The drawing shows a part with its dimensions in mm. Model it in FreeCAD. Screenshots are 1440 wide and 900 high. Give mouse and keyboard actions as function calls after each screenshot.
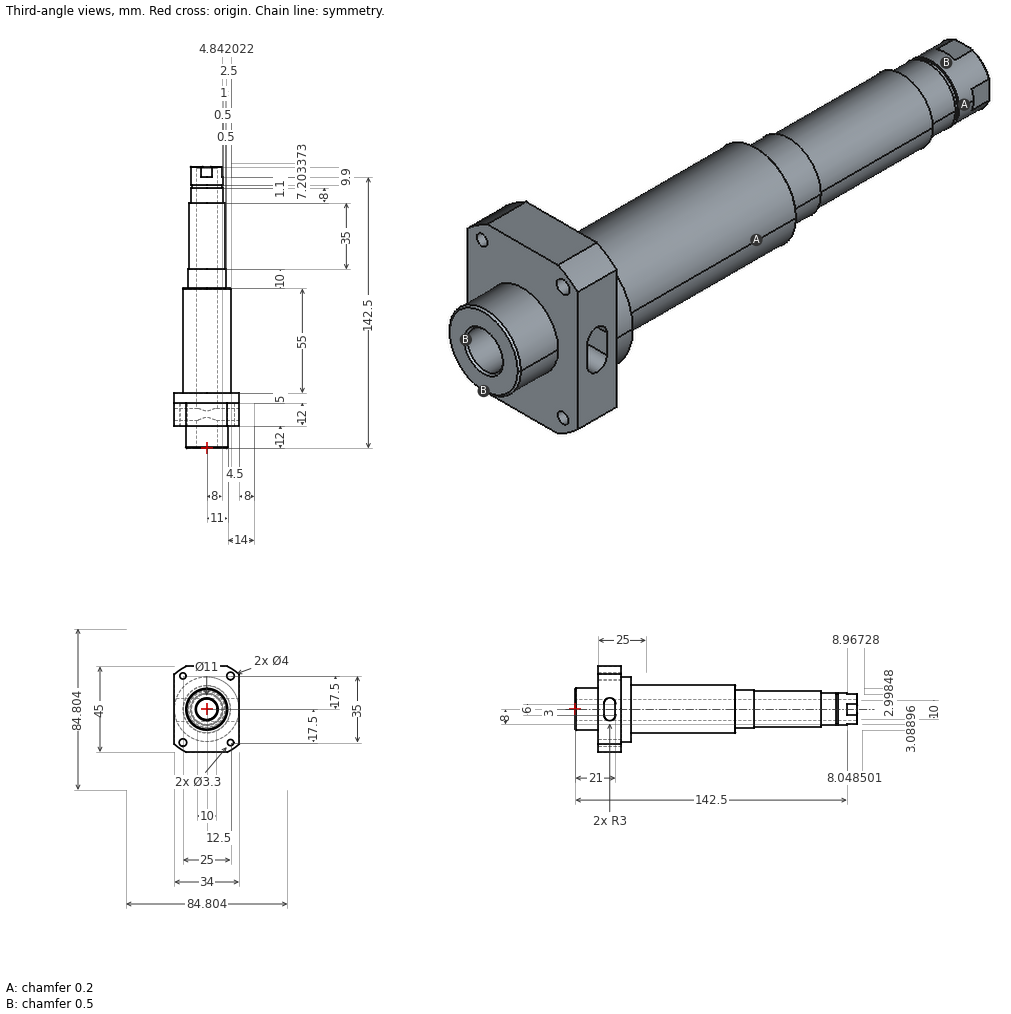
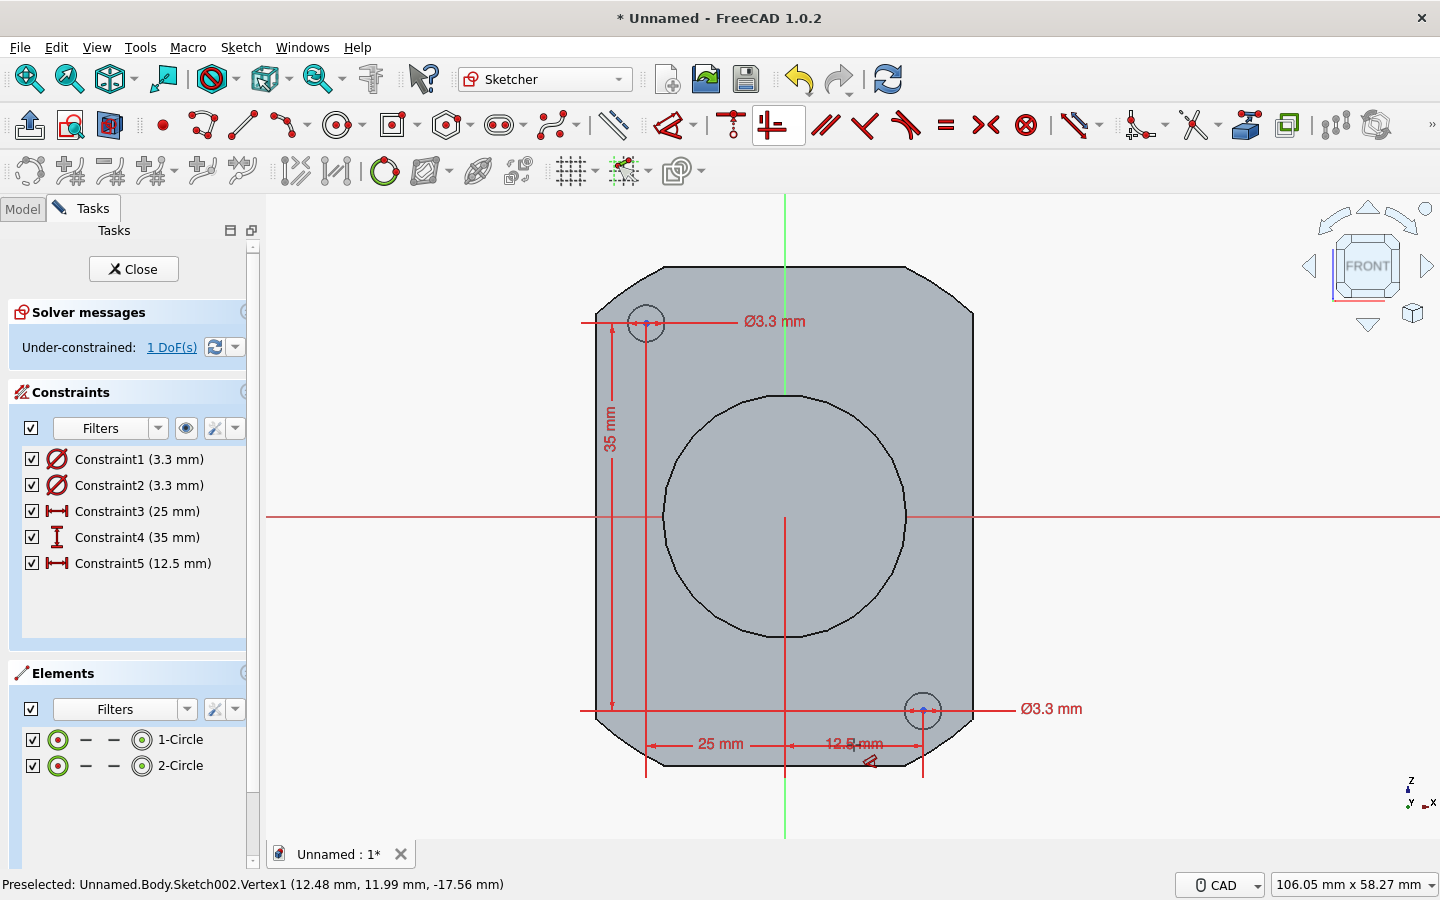
click(923, 711)
click(957, 614)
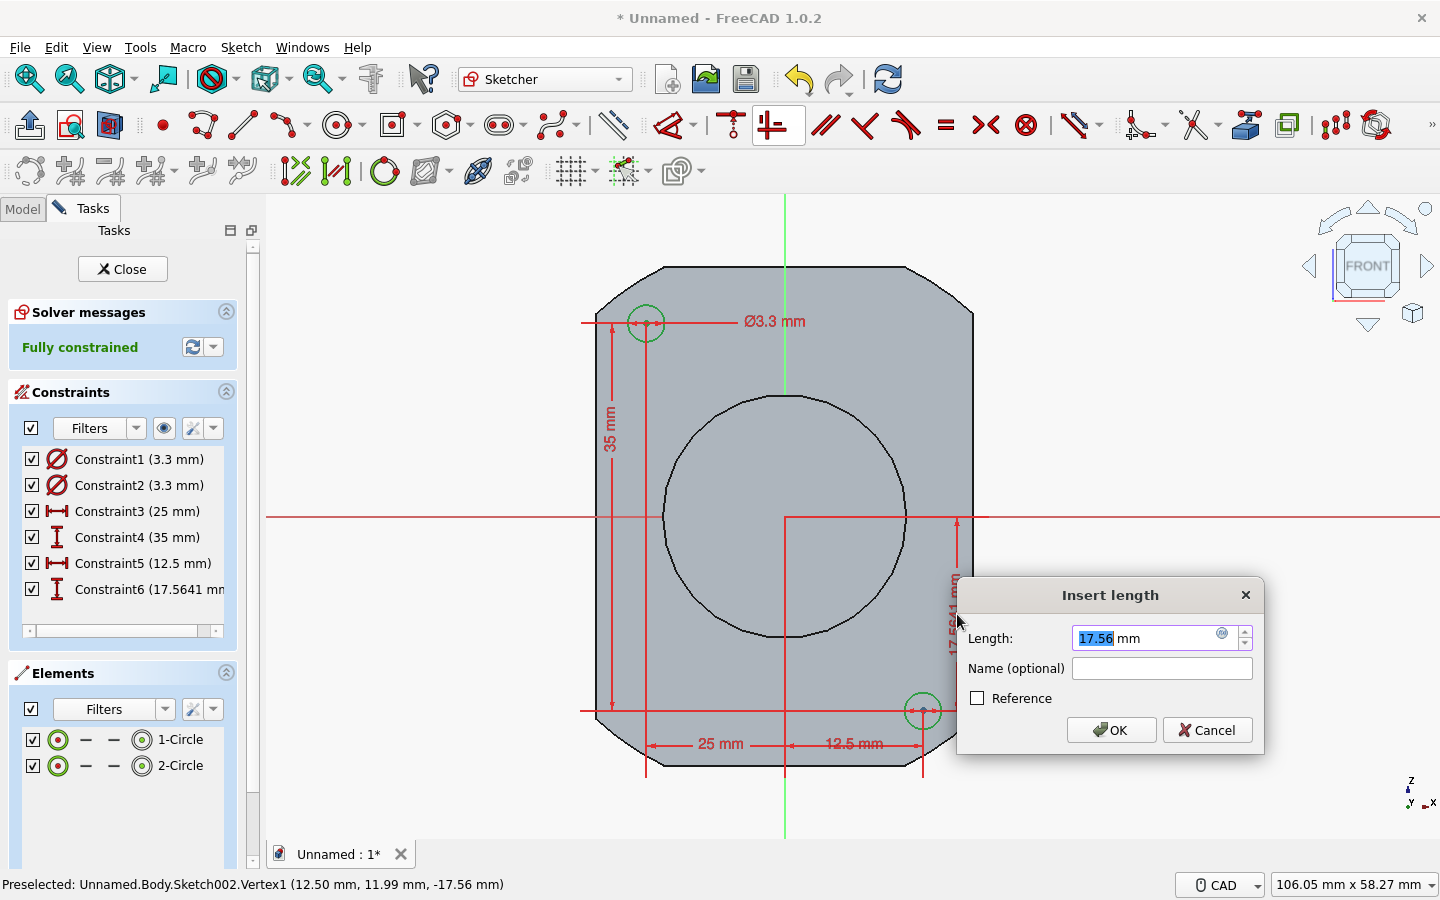
text(17.5)
key(Return)
key(Escape)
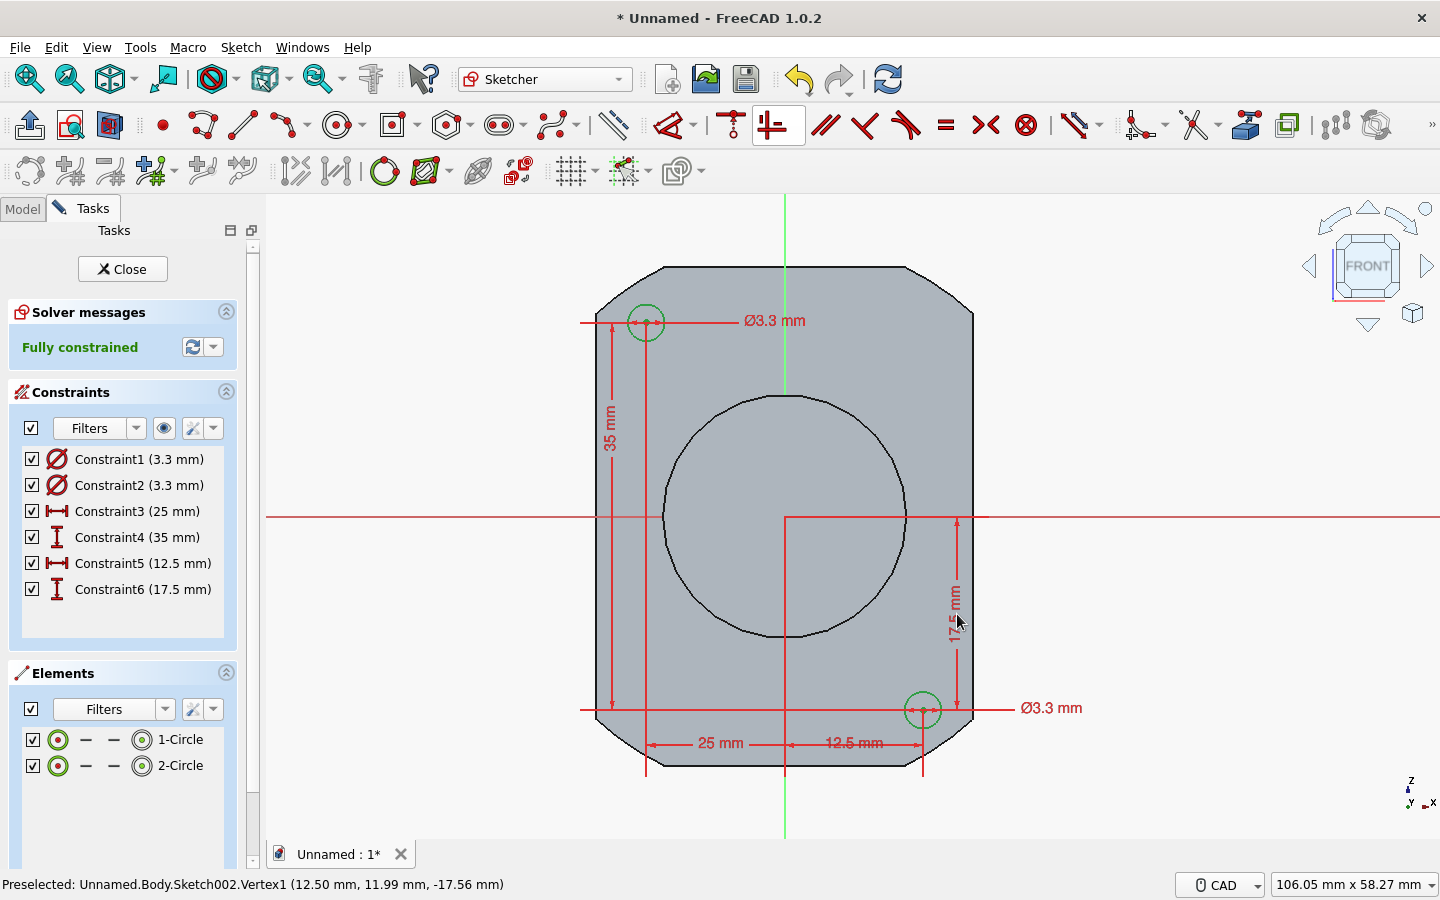
click(123, 269)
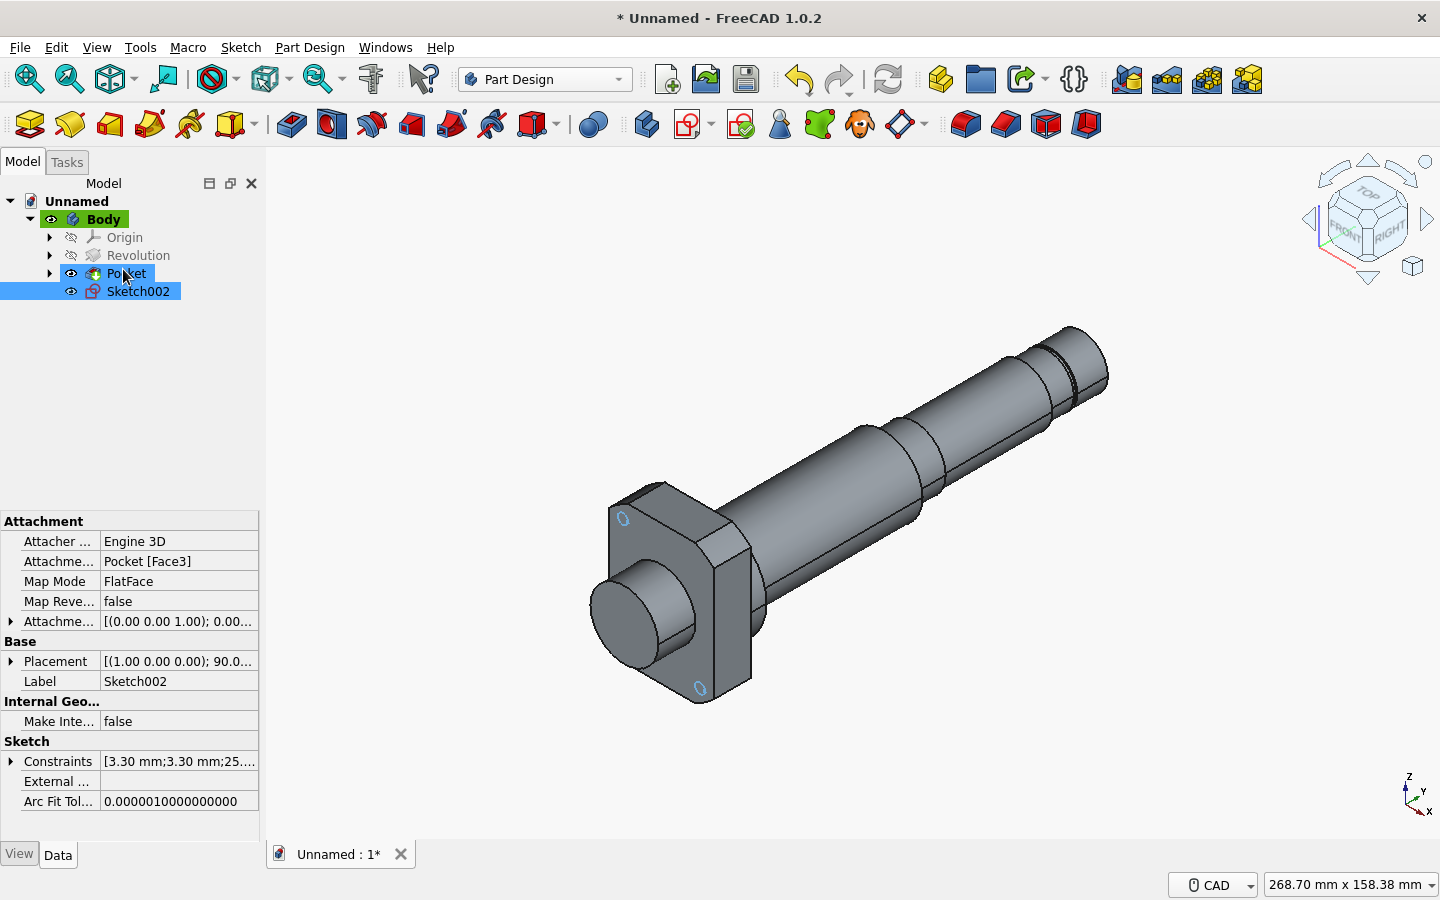
click(292, 124)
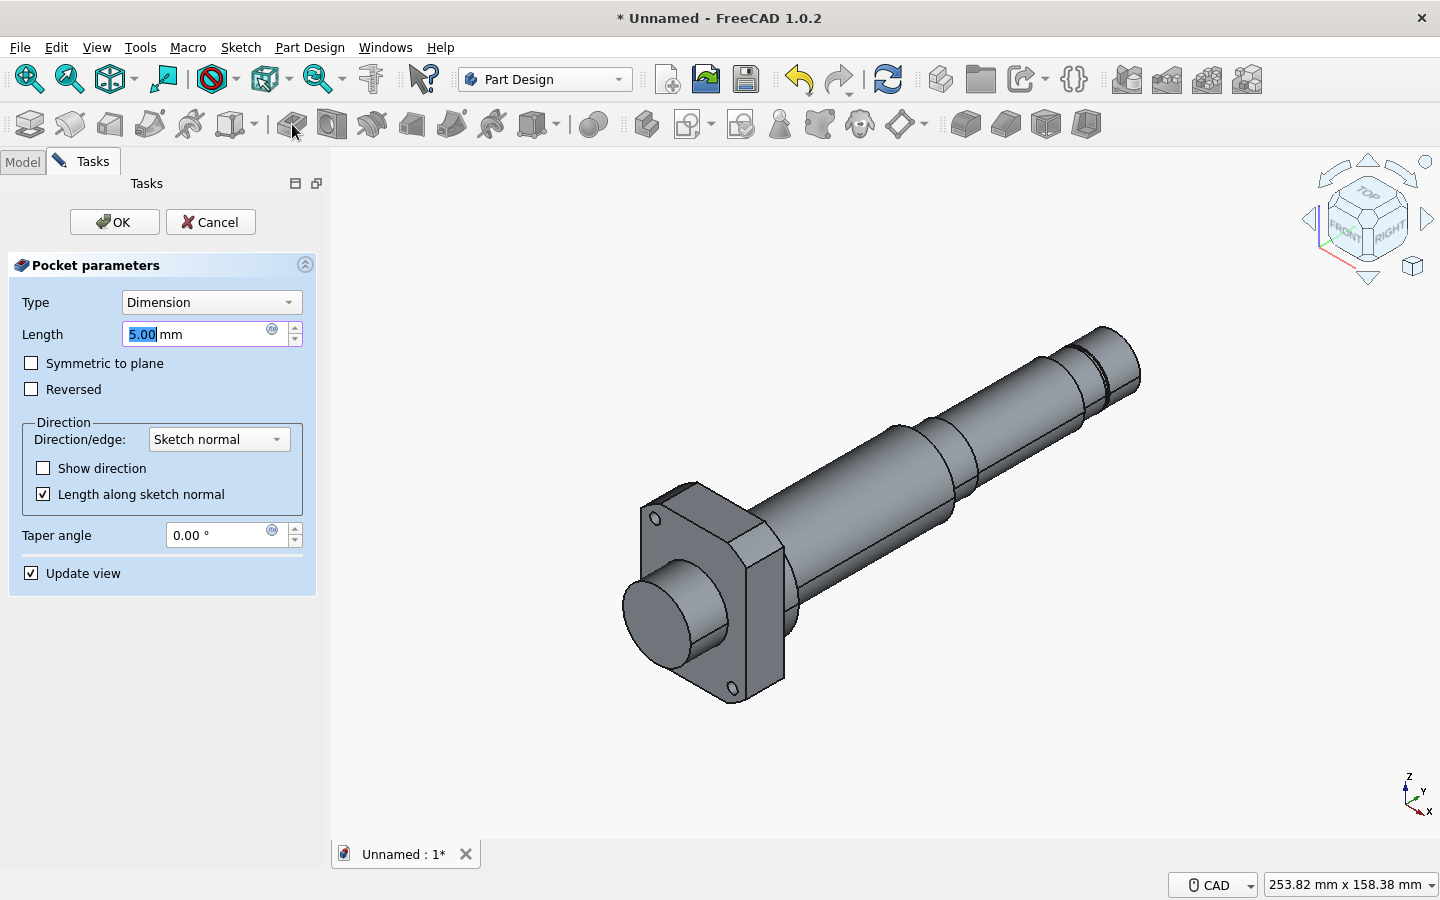
click(212, 302)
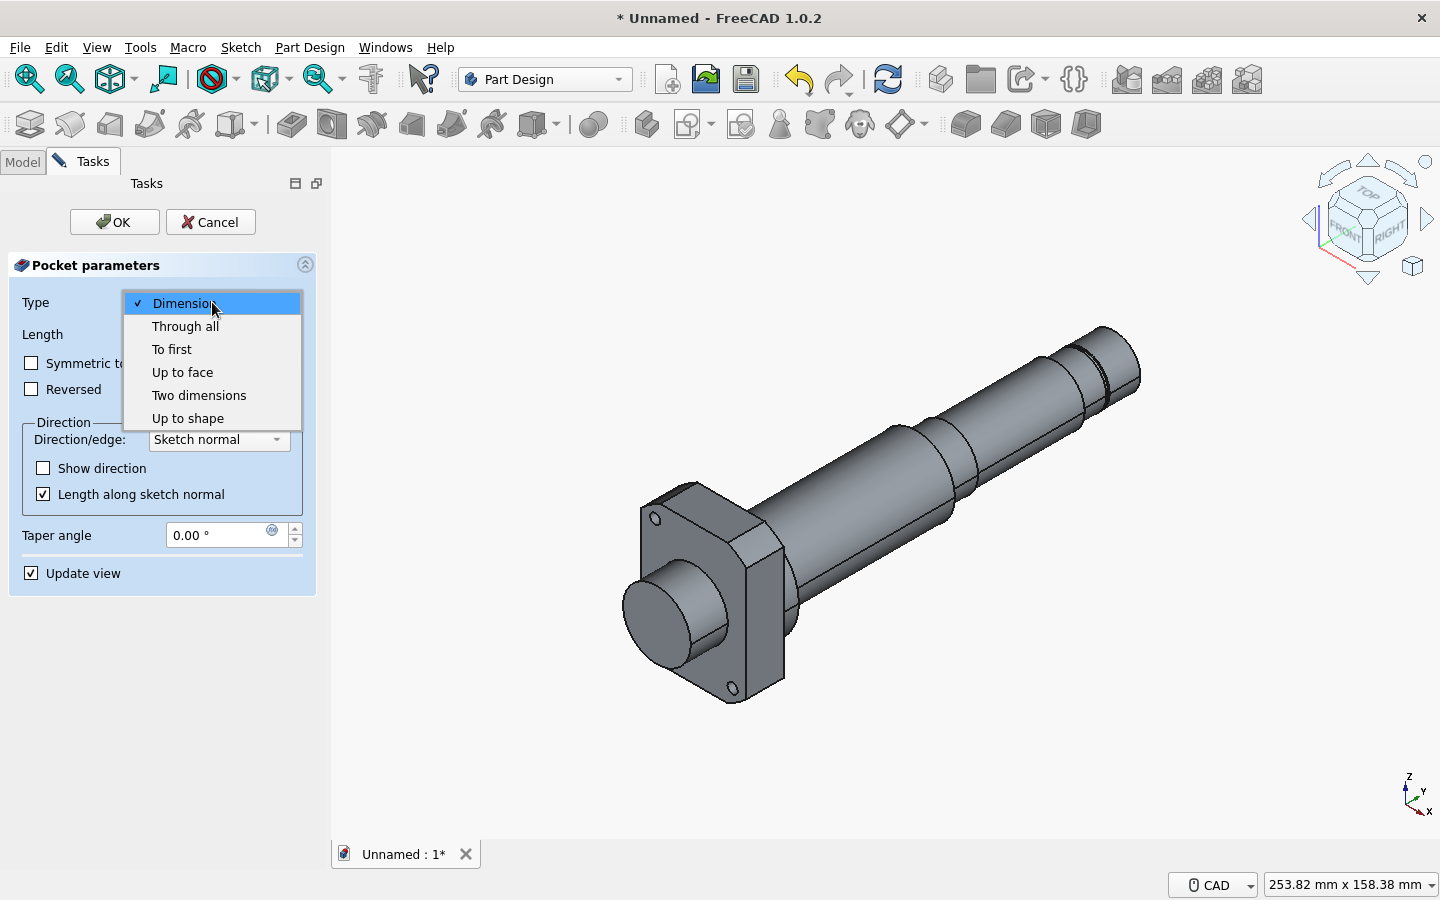
click(212, 326)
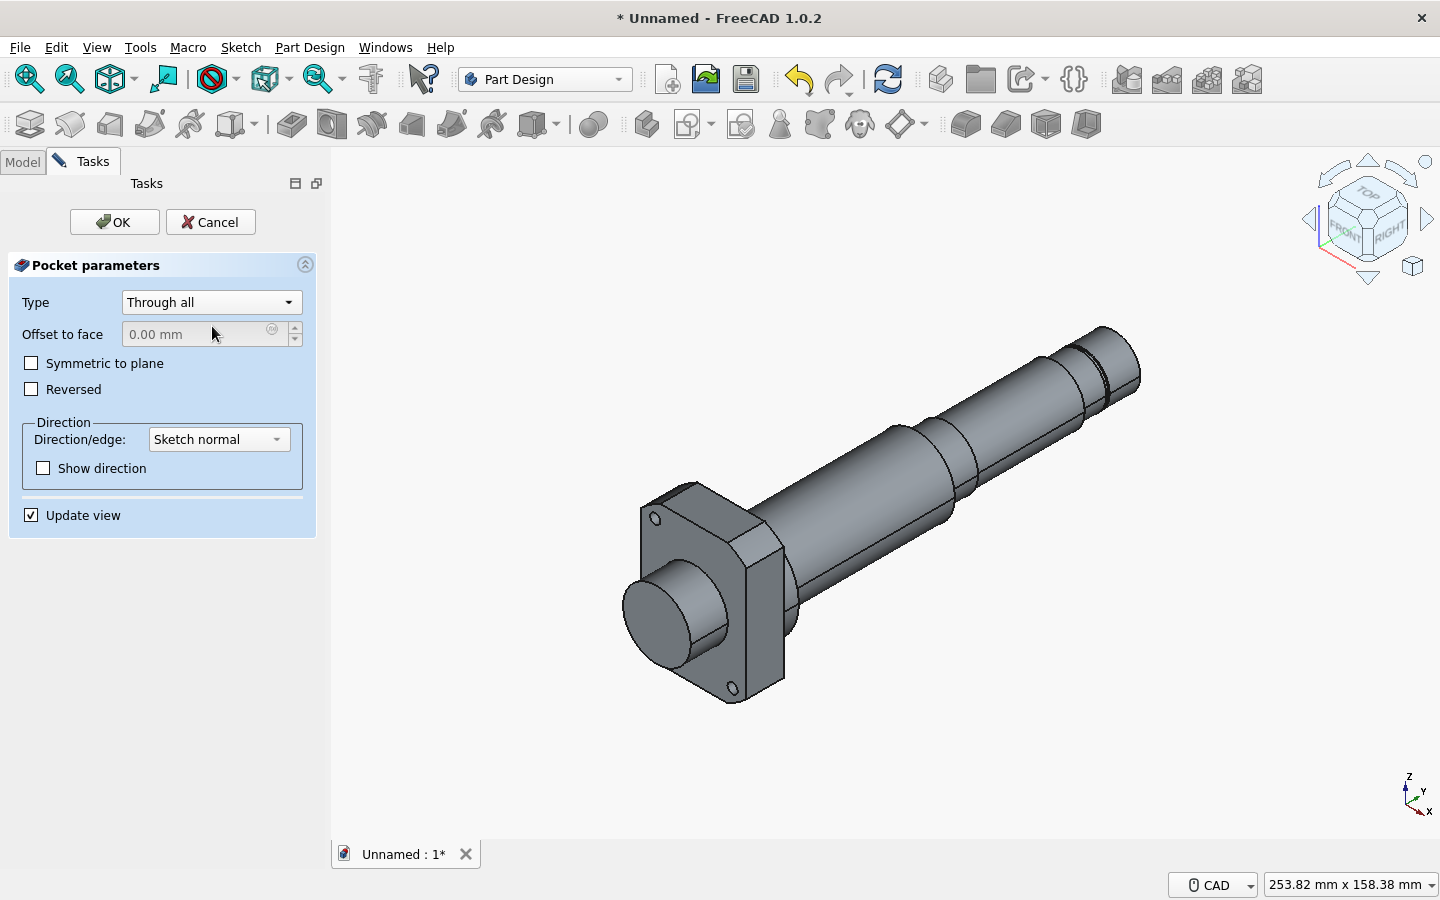
click(115, 222)